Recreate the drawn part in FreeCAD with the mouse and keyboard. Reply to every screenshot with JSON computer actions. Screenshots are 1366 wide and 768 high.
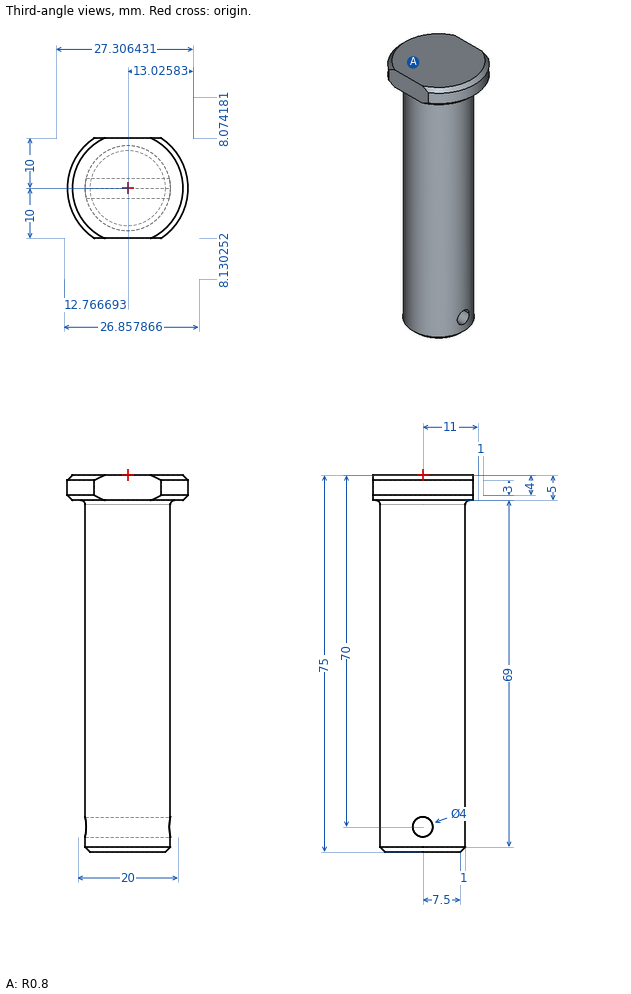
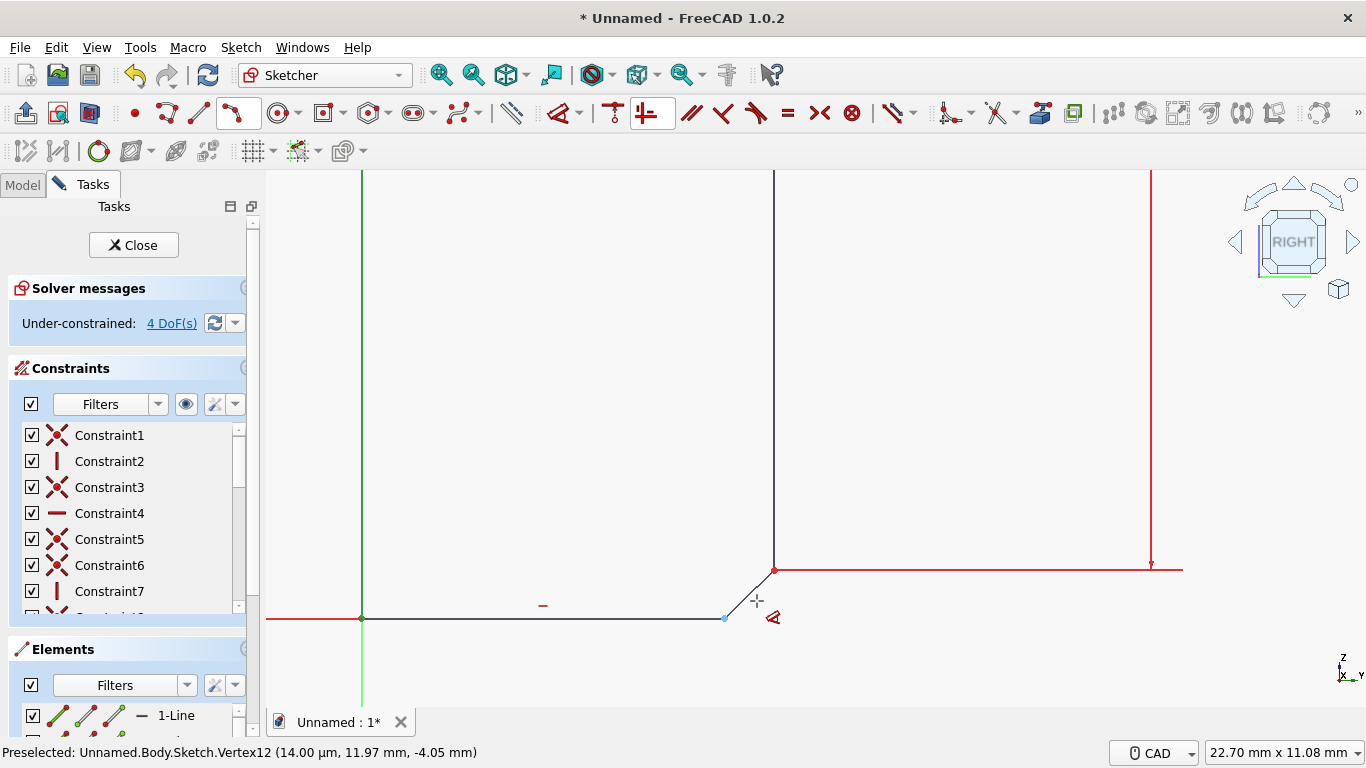
{"action": "left_click", "coordinate": [749, 595]}
{"action": "left_click", "coordinate": [749, 653]}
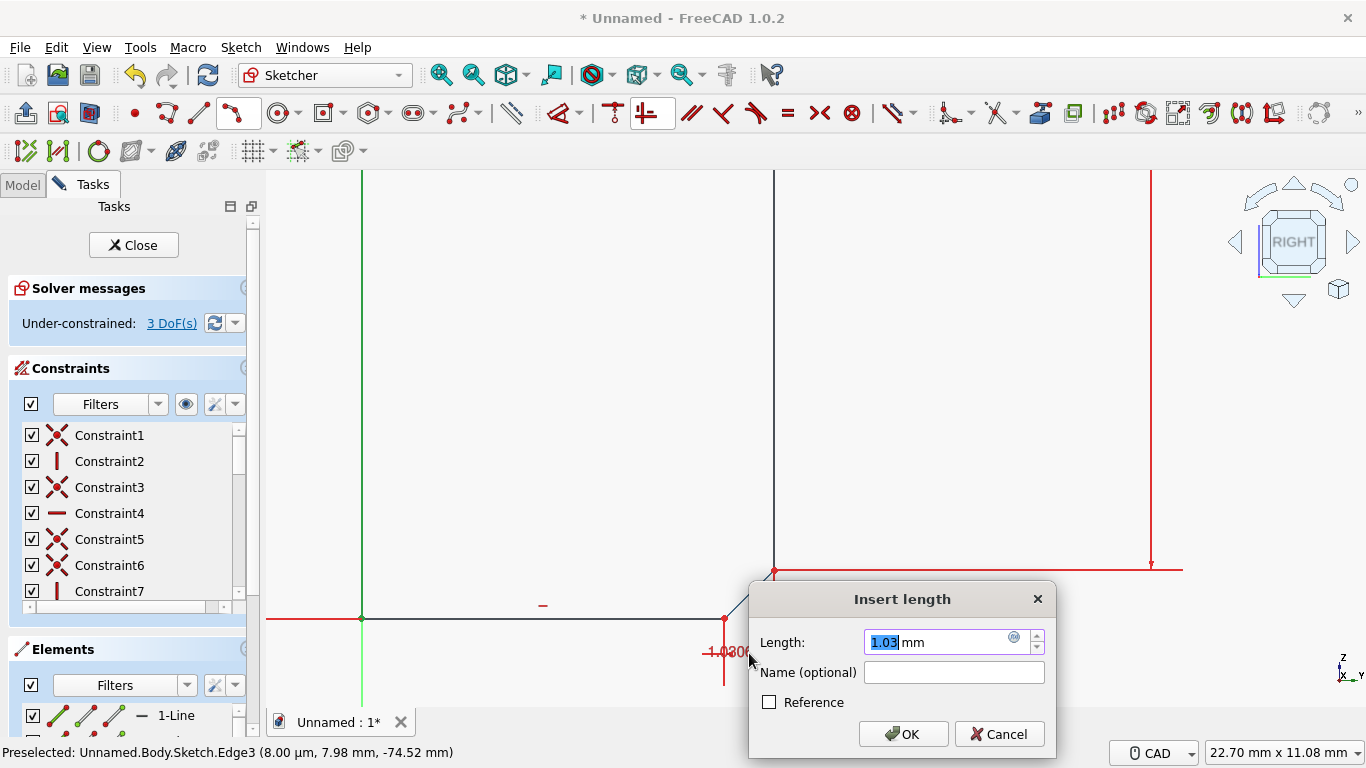
{"action": "type", "text": "1"}
{"action": "key", "text": "Return"}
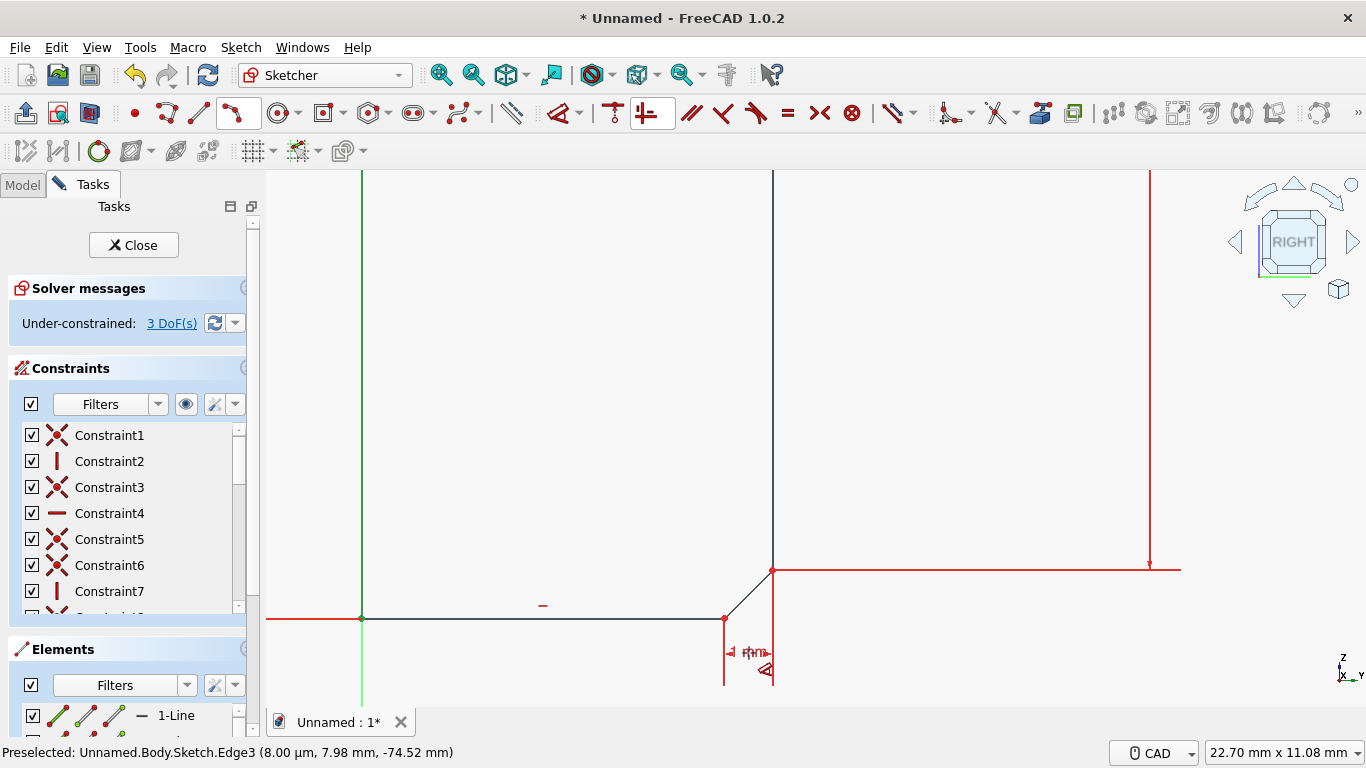
{"action": "scroll", "coordinate": [757, 602], "scroll_direction": "down", "scroll_amount": 12}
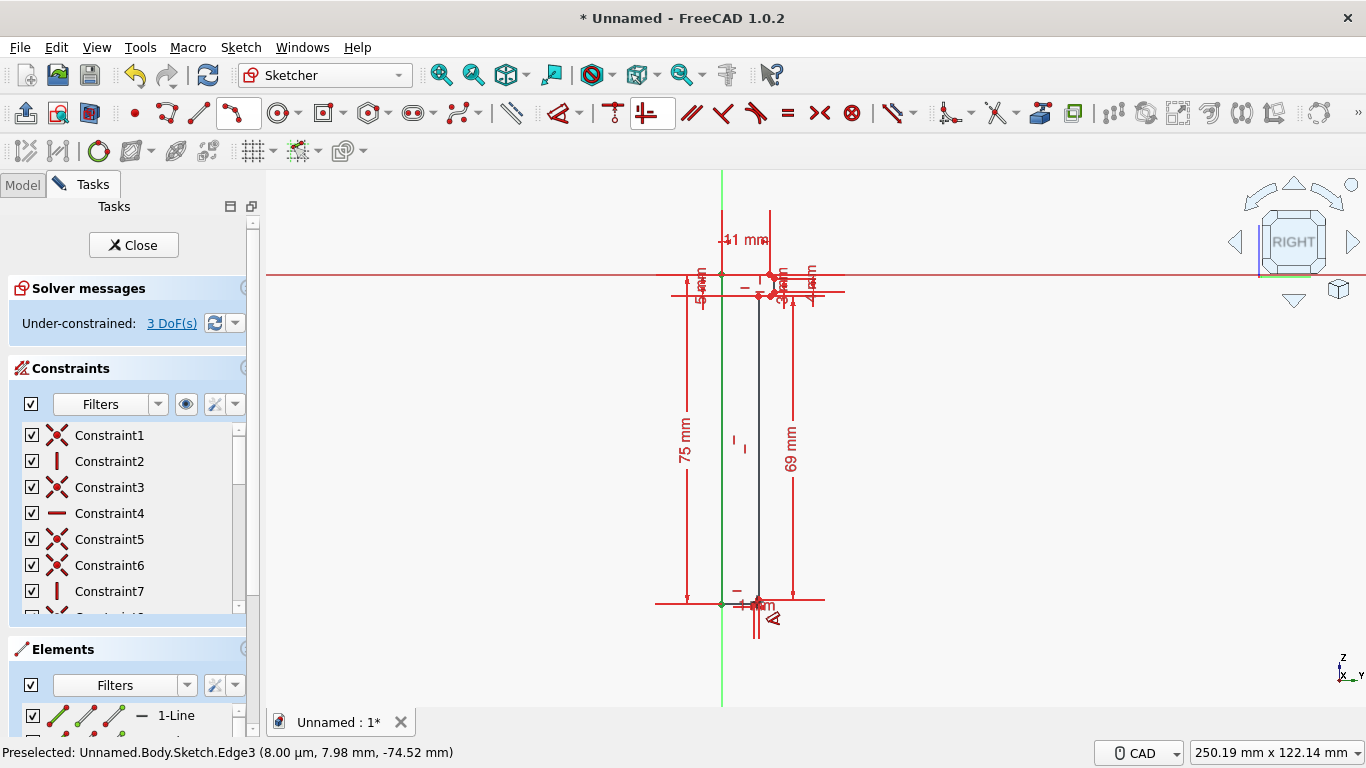
{"action": "scroll", "coordinate": [771, 295], "scroll_direction": "up", "scroll_amount": 12}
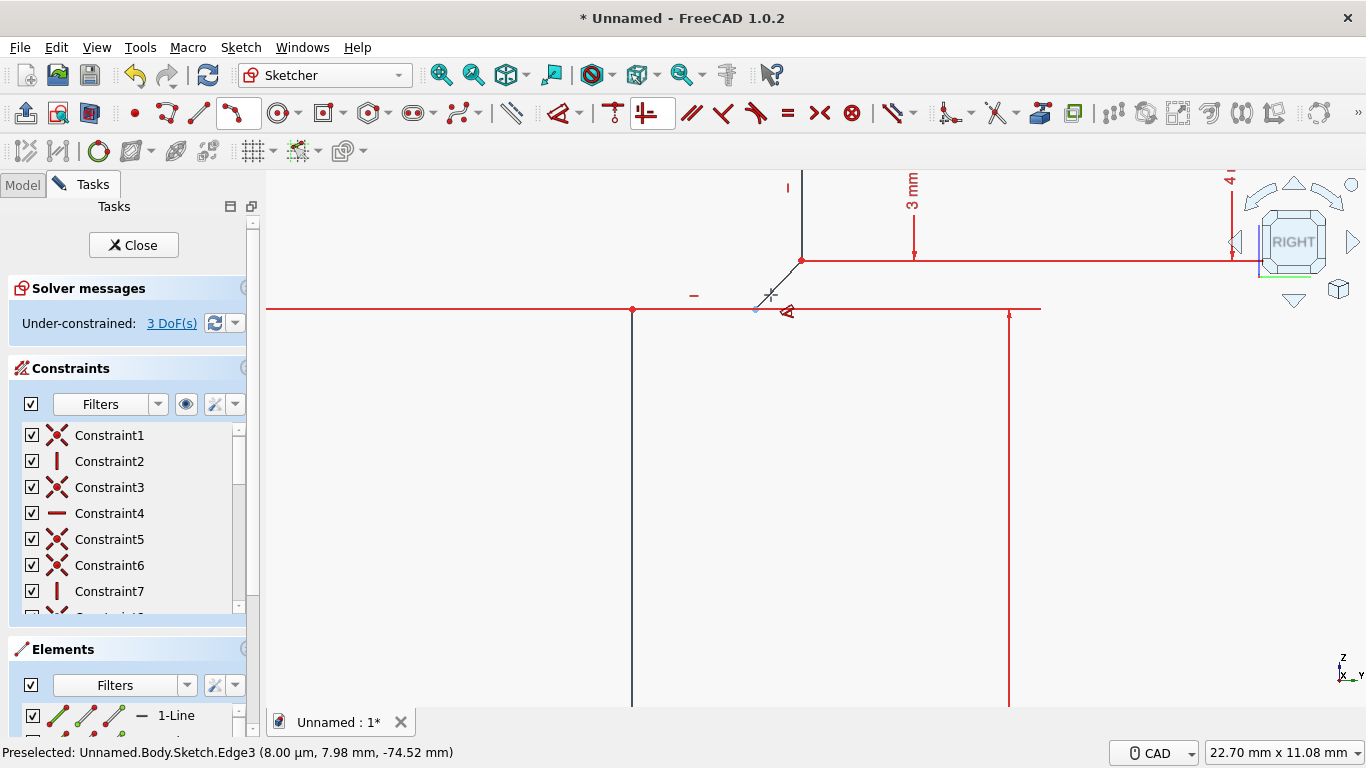
{"action": "left_click", "coordinate": [770, 295]}
{"action": "left_click", "coordinate": [779, 227]}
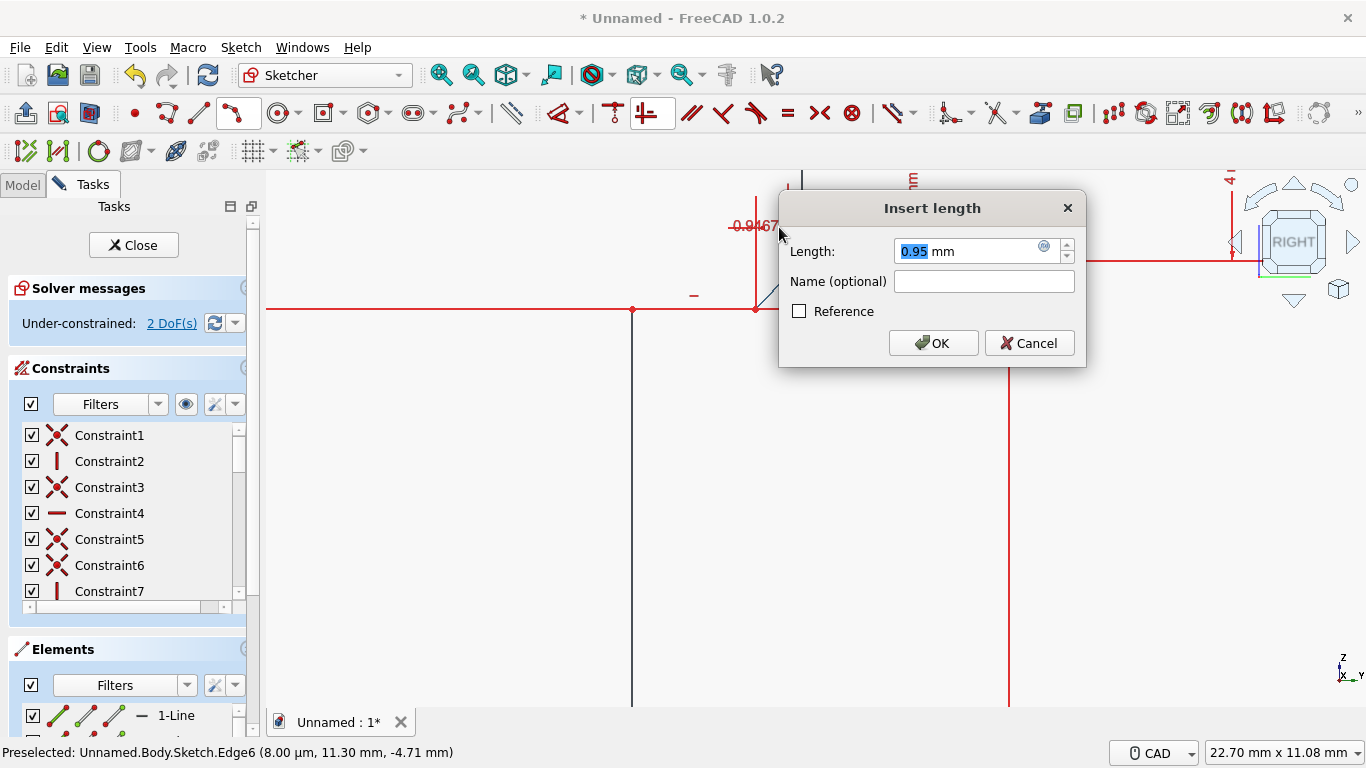
{"action": "type", "text": "1"}
{"action": "key", "text": "Return"}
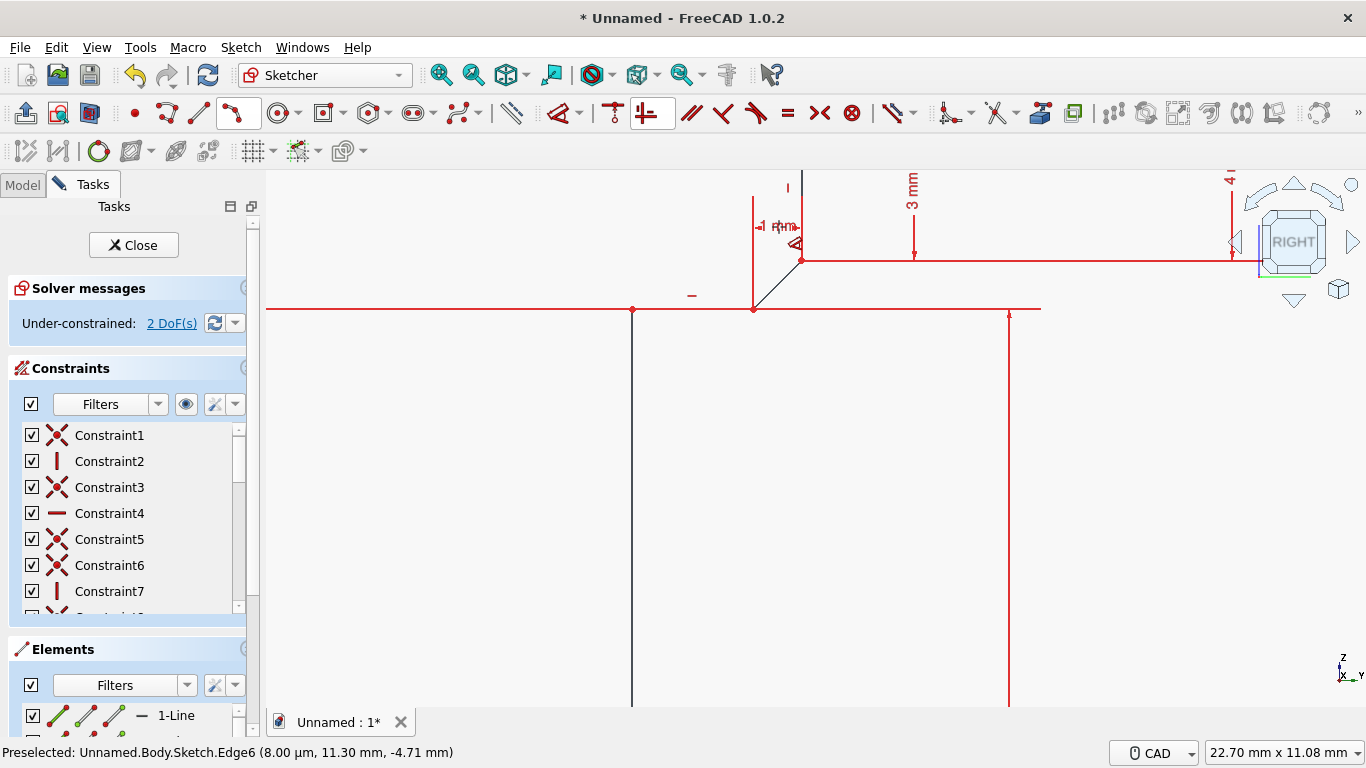
{"action": "scroll", "coordinate": [771, 294], "scroll_direction": "down", "scroll_amount": 12}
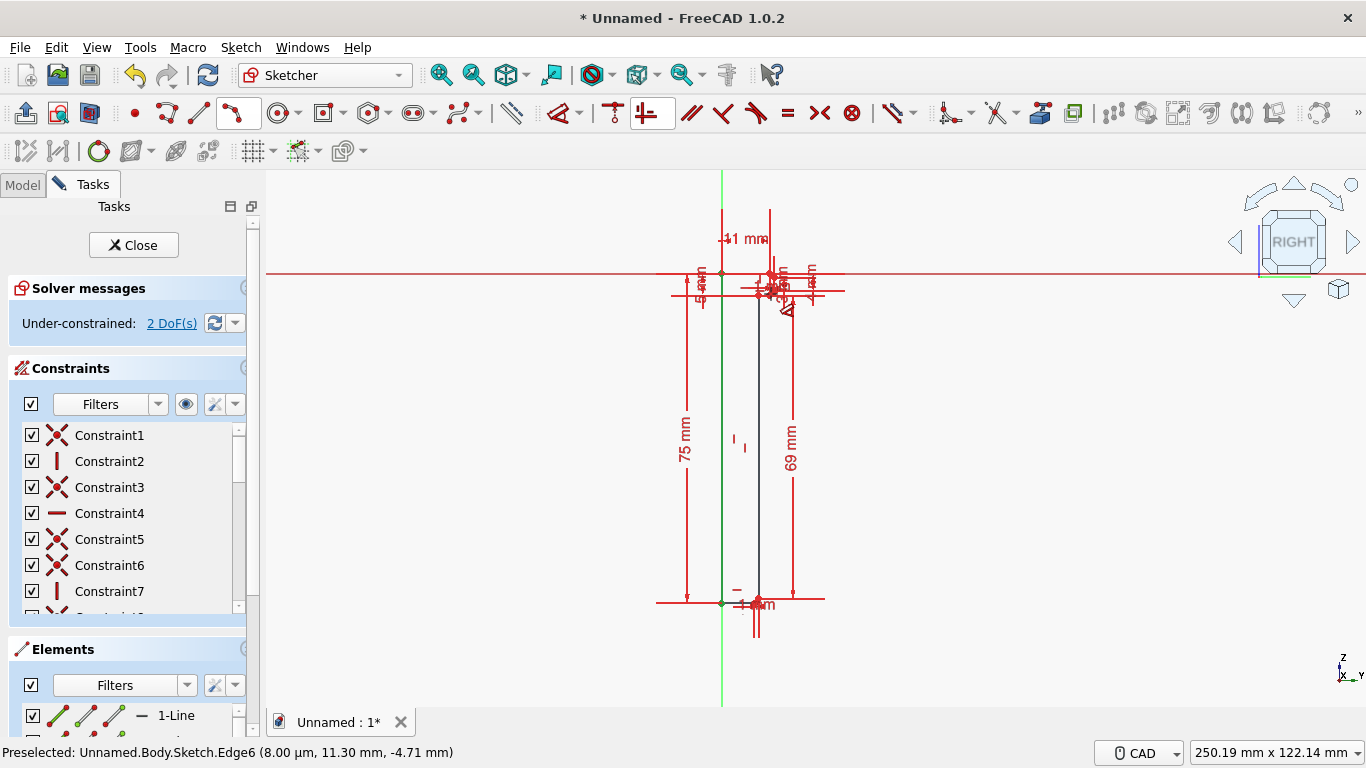
{"action": "scroll", "coordinate": [773, 277], "scroll_direction": "up", "scroll_amount": 12}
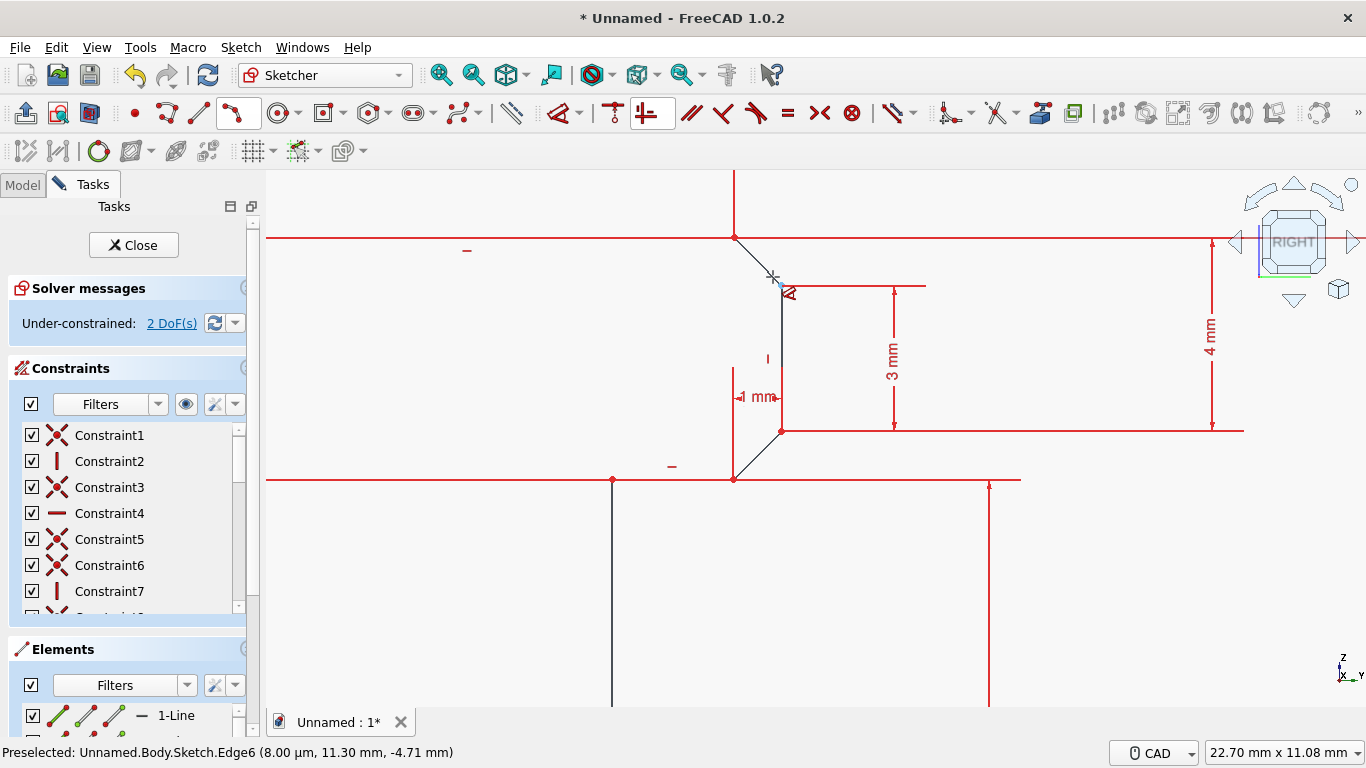
{"action": "left_click", "coordinate": [767, 271]}
{"action": "left_click", "coordinate": [758, 204]}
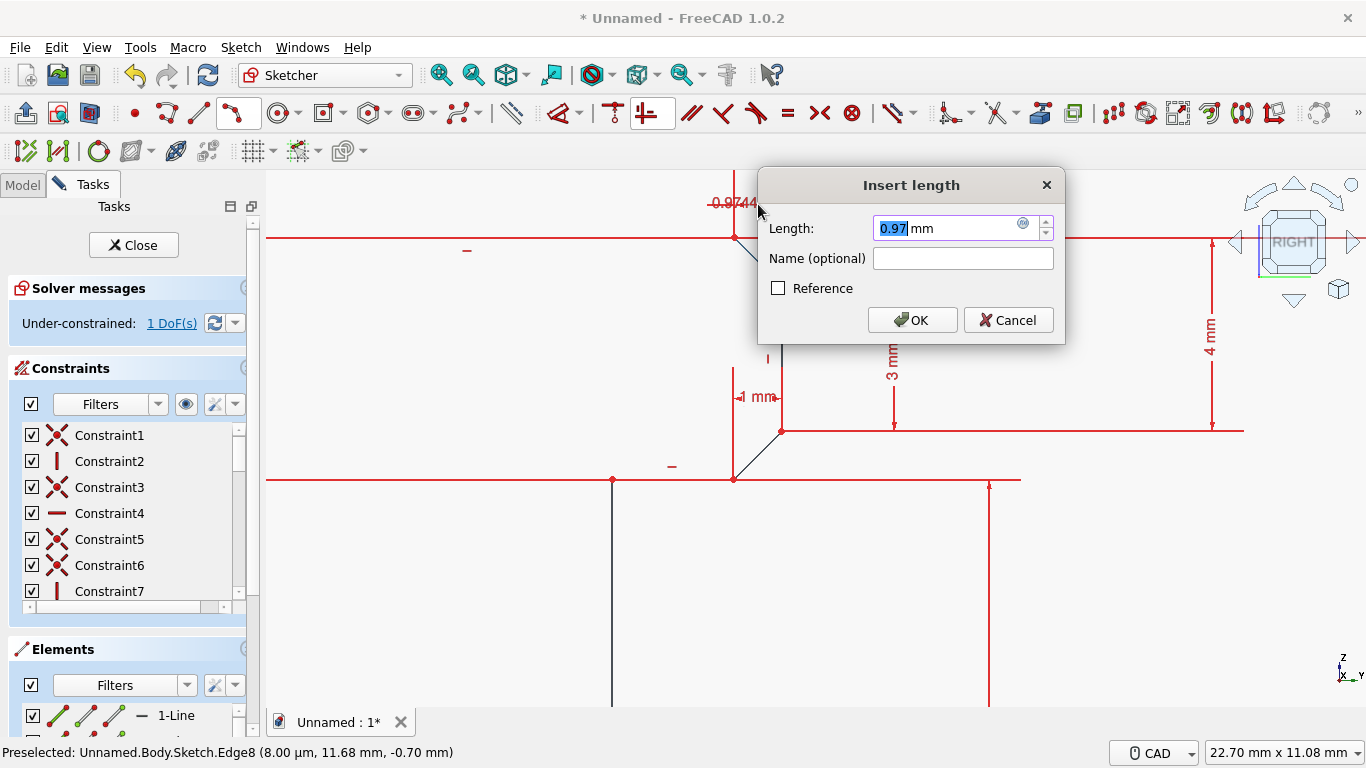
{"action": "type", "text": "1"}
{"action": "key", "text": "Return"}